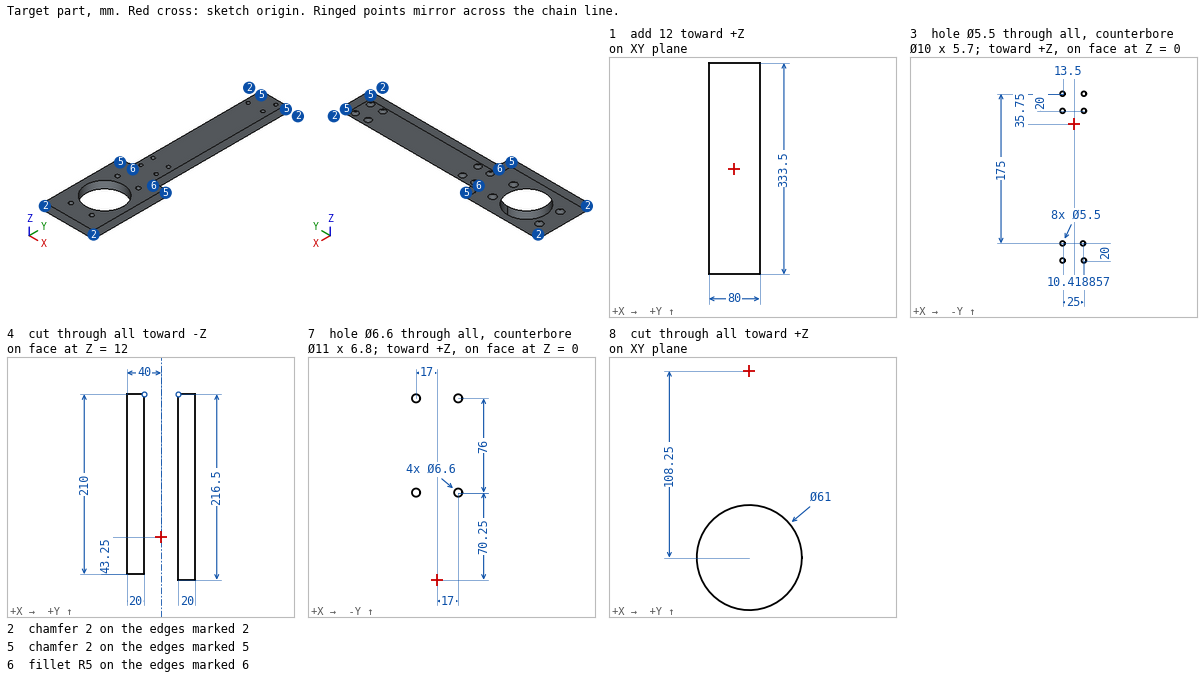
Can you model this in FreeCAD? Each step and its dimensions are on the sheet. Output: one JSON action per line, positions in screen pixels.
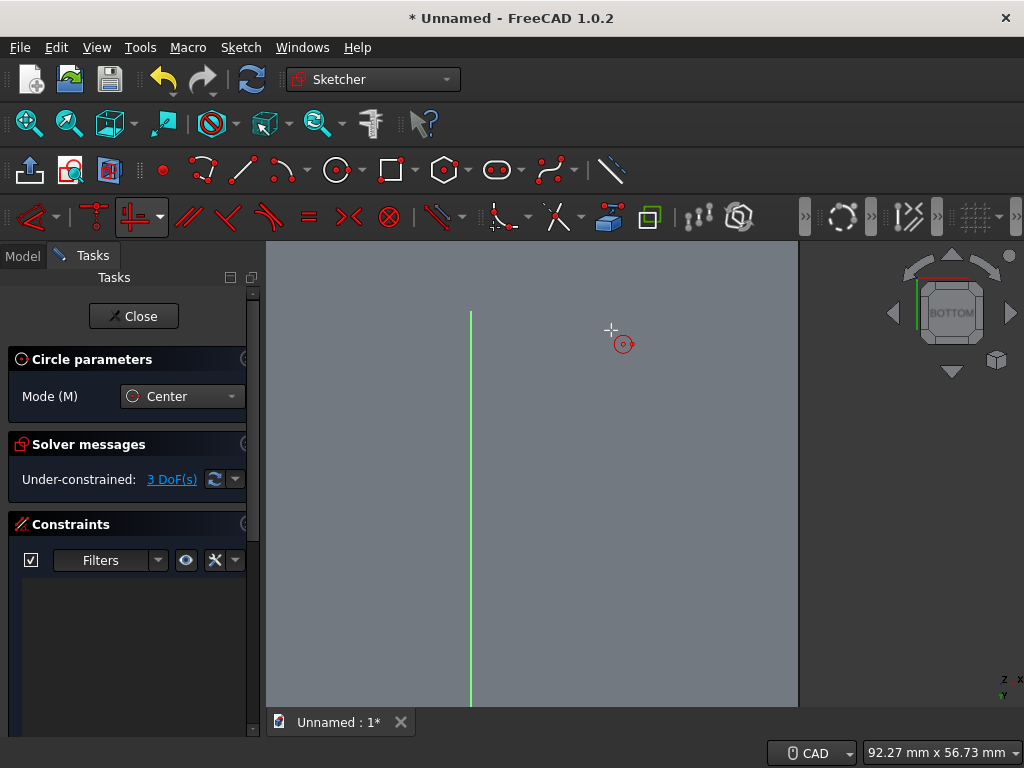
{"action": "scroll", "coordinate": [611, 329], "scroll_direction": "down", "scroll_amount": 7}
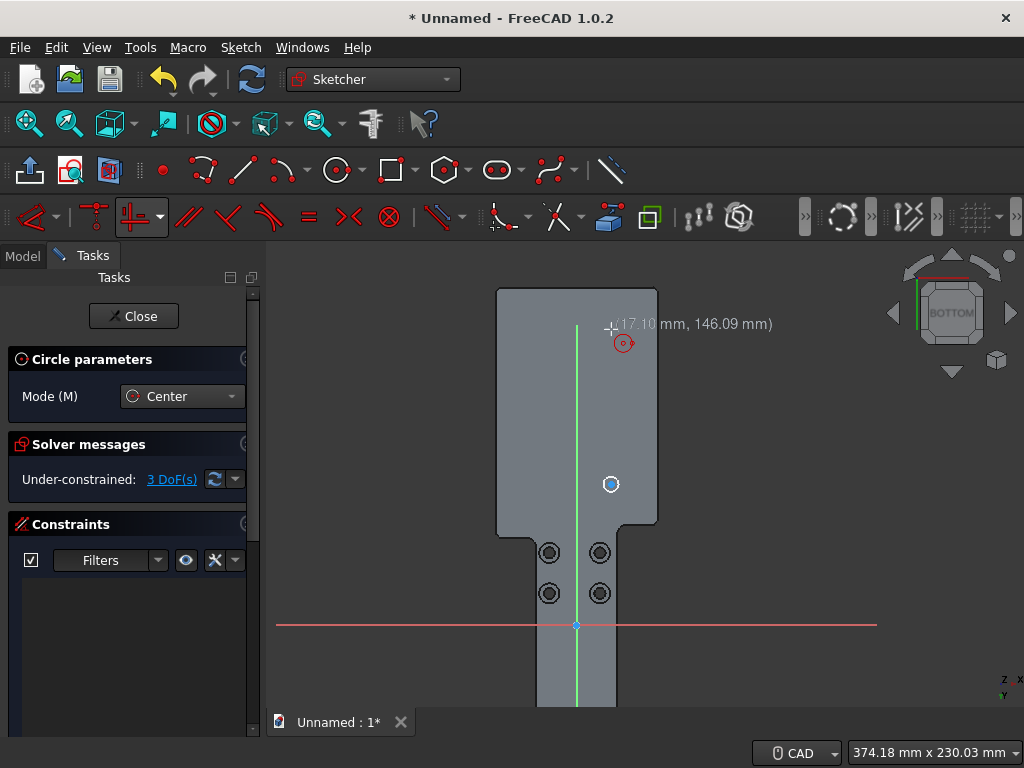
{"action": "left_click", "coordinate": [611, 329]}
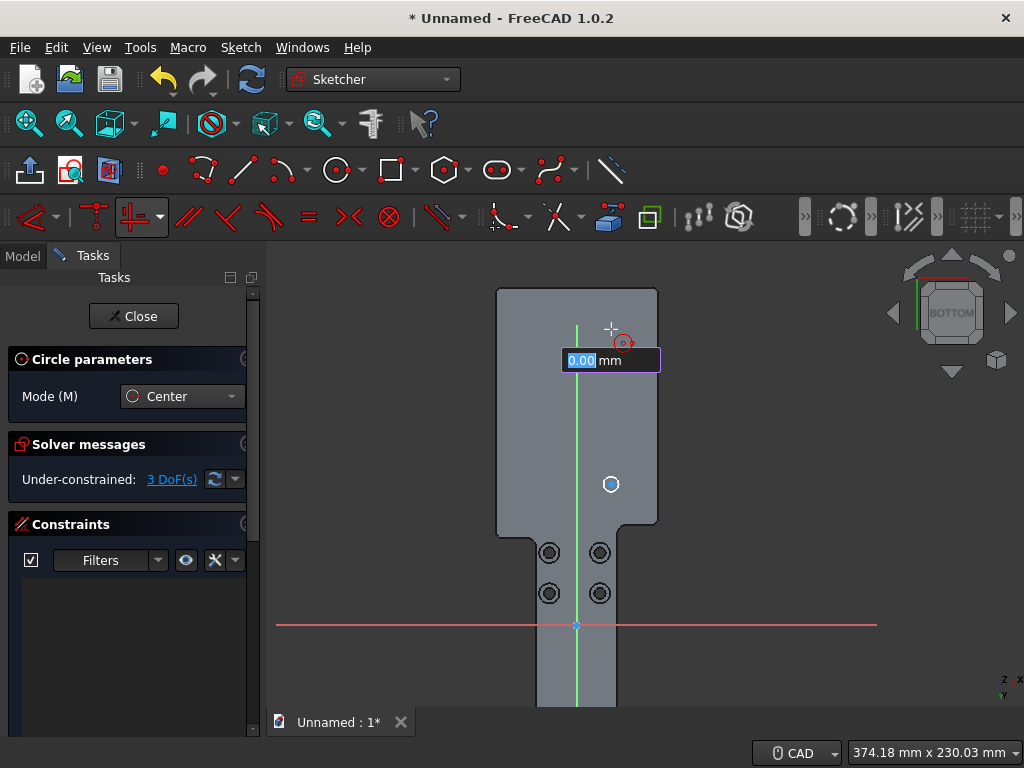
{"action": "scroll", "coordinate": [616, 324], "scroll_direction": "up", "scroll_amount": 5}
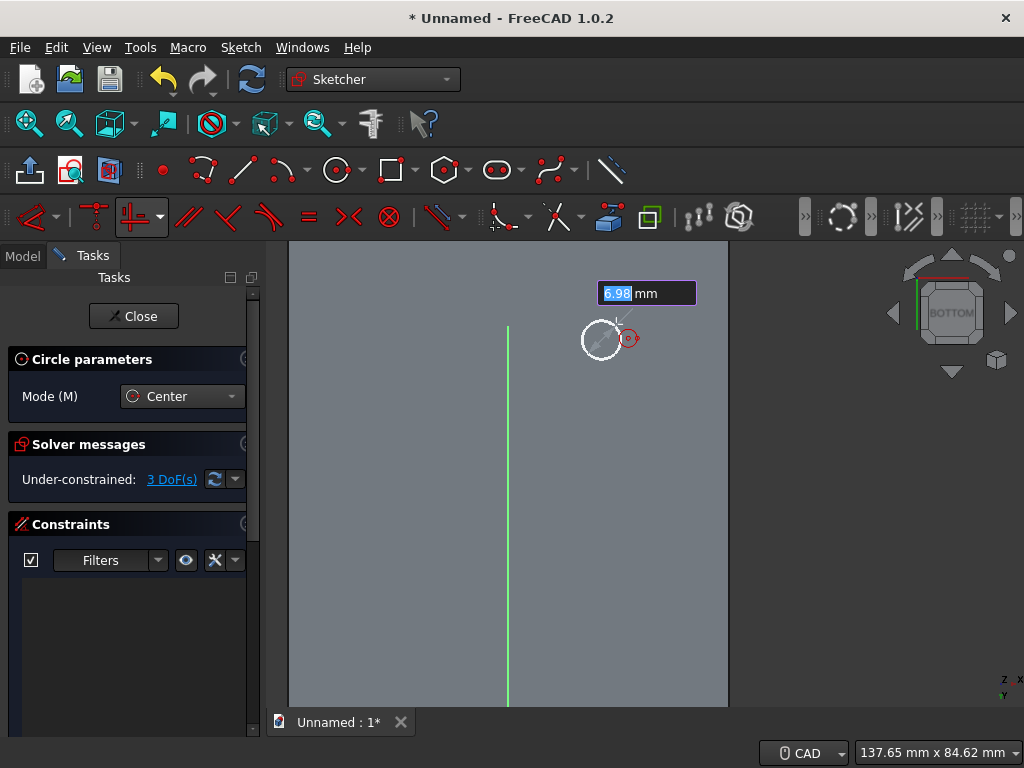
{"action": "left_click", "coordinate": [615, 325]}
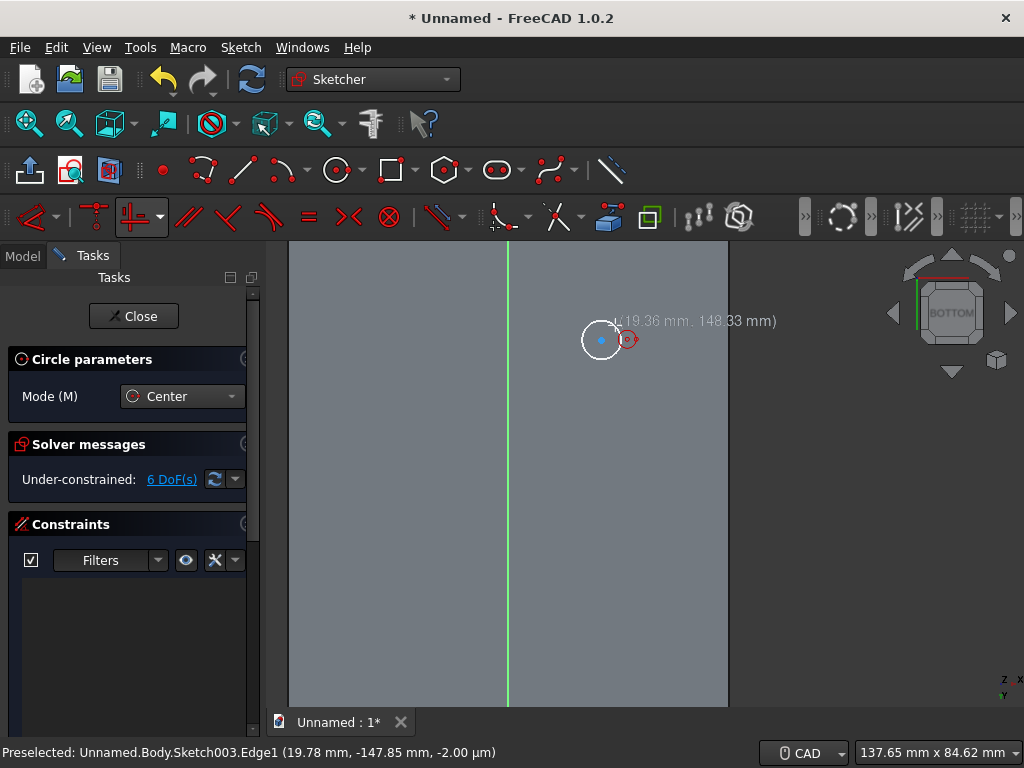
{"action": "scroll", "coordinate": [415, 337], "scroll_direction": "up", "scroll_amount": 2}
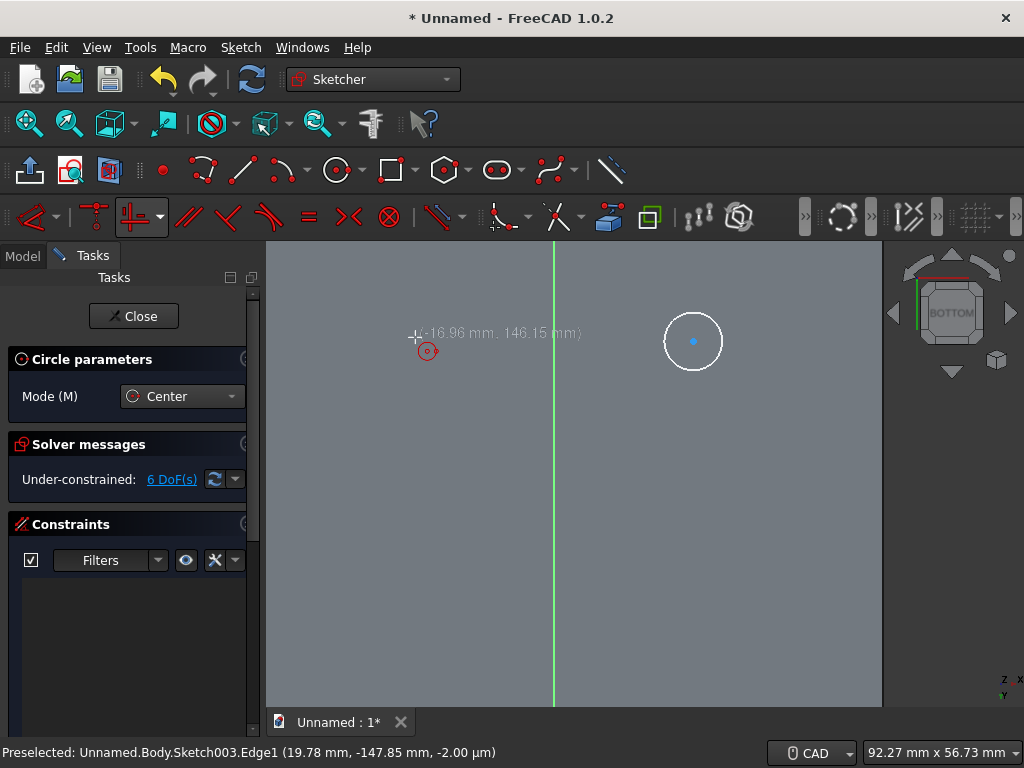
{"action": "scroll", "coordinate": [584, 326], "scroll_direction": "down", "scroll_amount": 7}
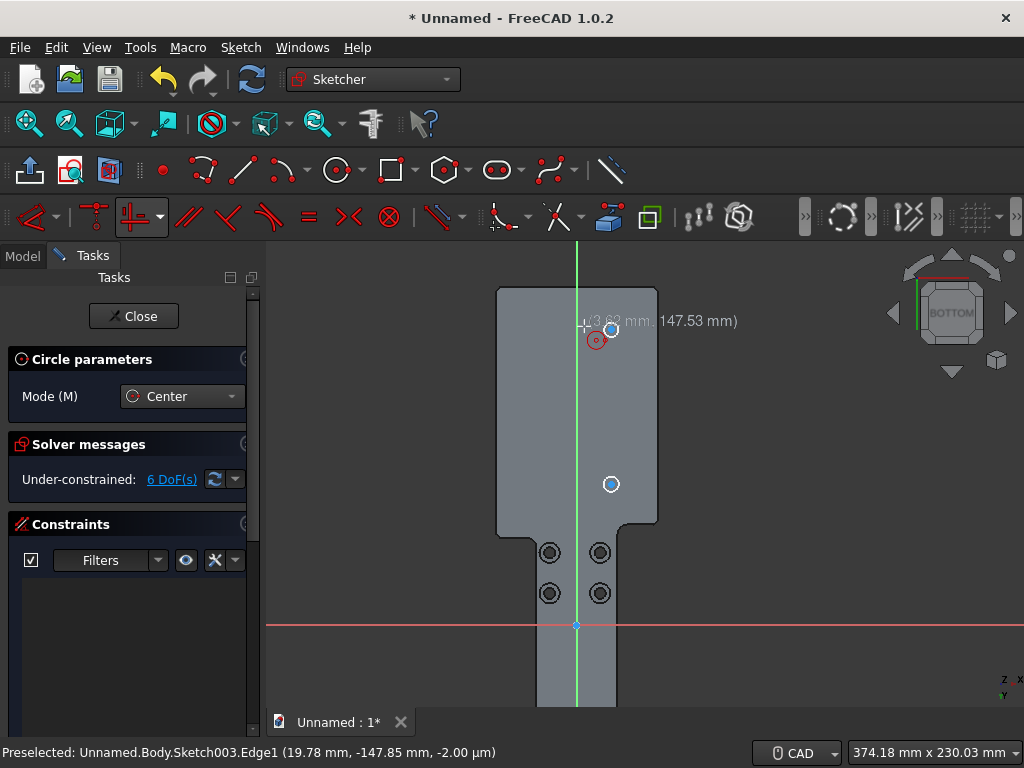
{"action": "left_click", "coordinate": [543, 329]}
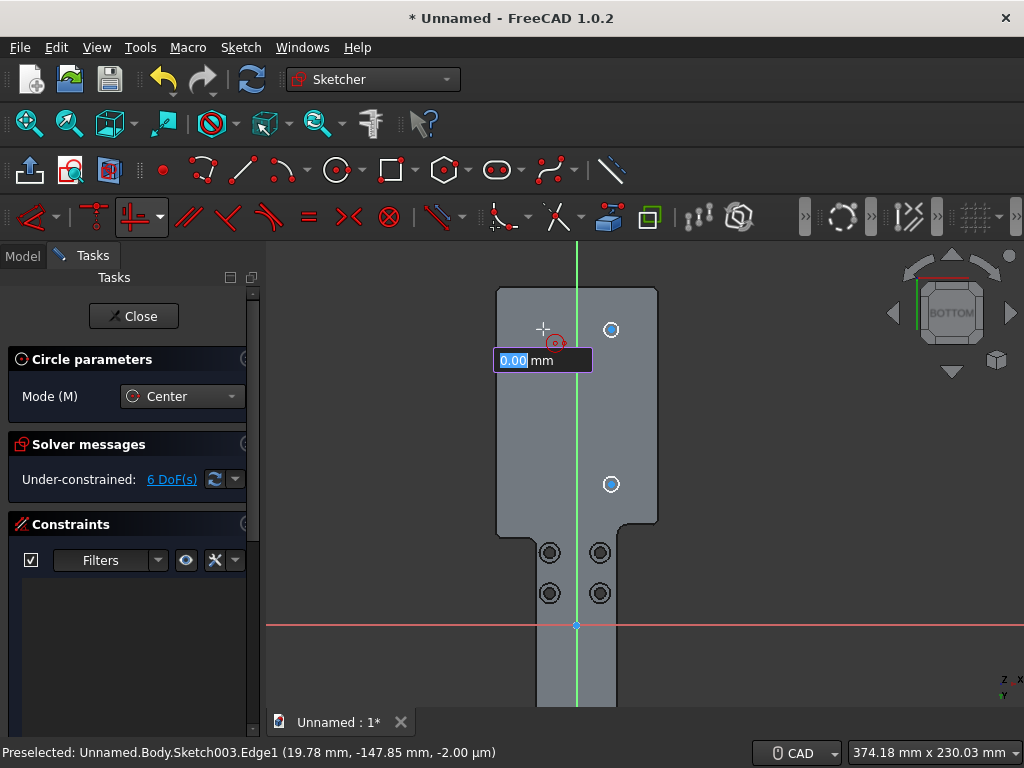
{"action": "scroll", "coordinate": [547, 324], "scroll_direction": "up", "scroll_amount": 5}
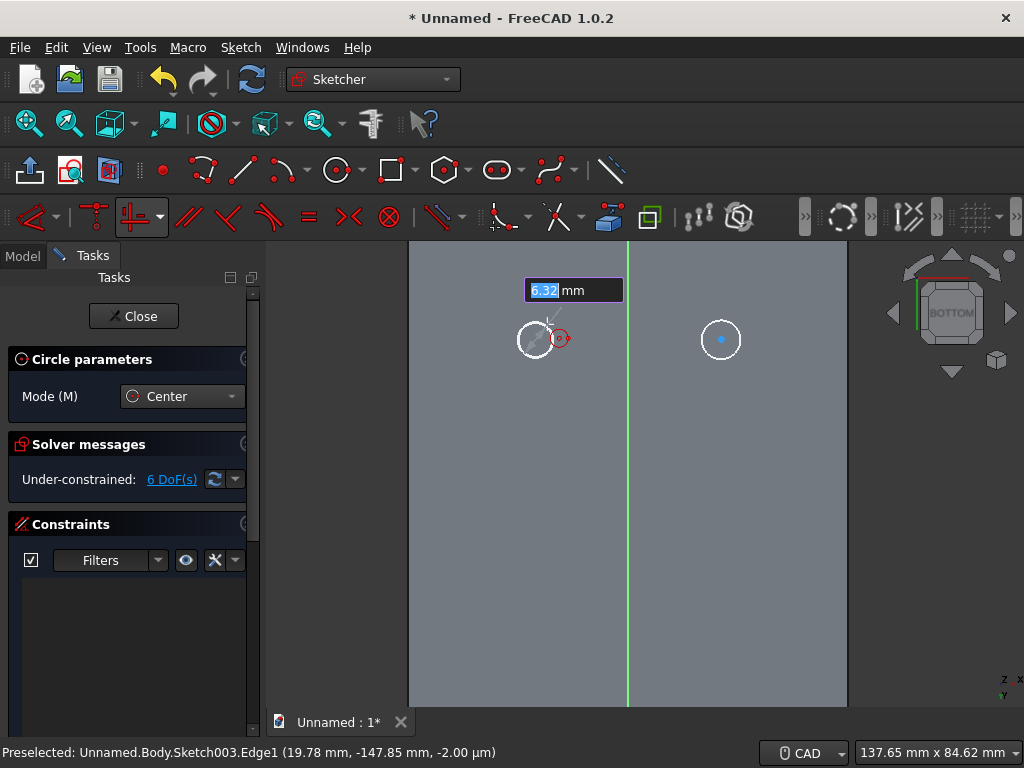
{"action": "left_click", "coordinate": [547, 324]}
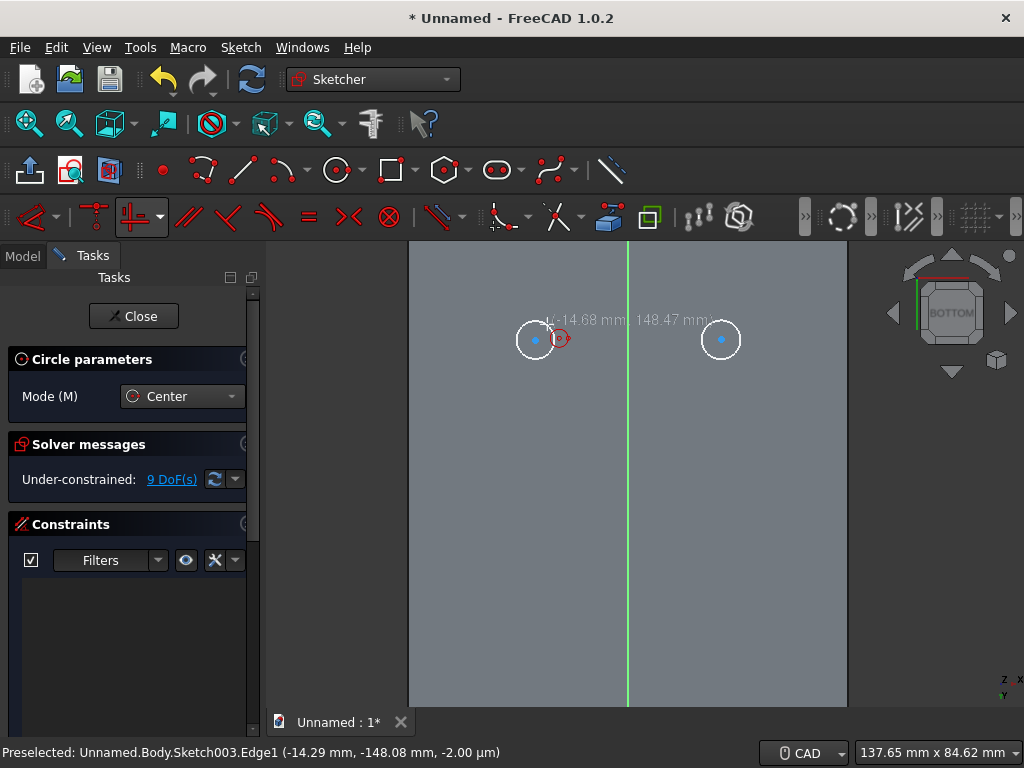
{"action": "scroll", "coordinate": [547, 325], "scroll_direction": "down", "scroll_amount": 5}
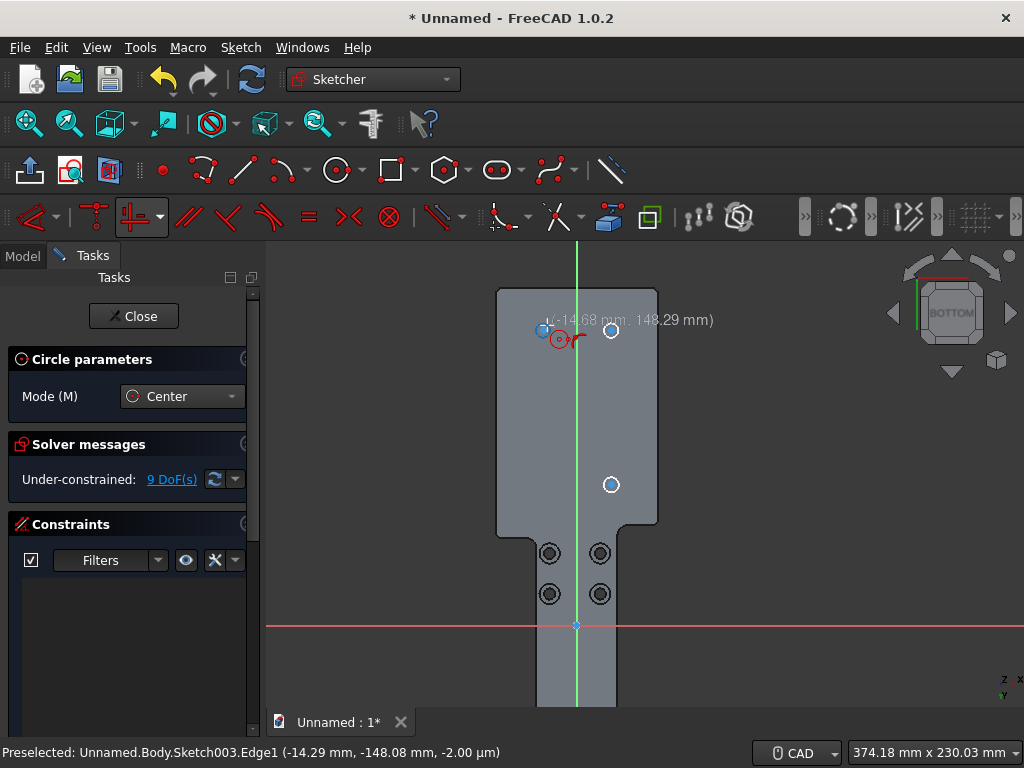
{"action": "scroll", "coordinate": [543, 484], "scroll_direction": "up", "scroll_amount": 7}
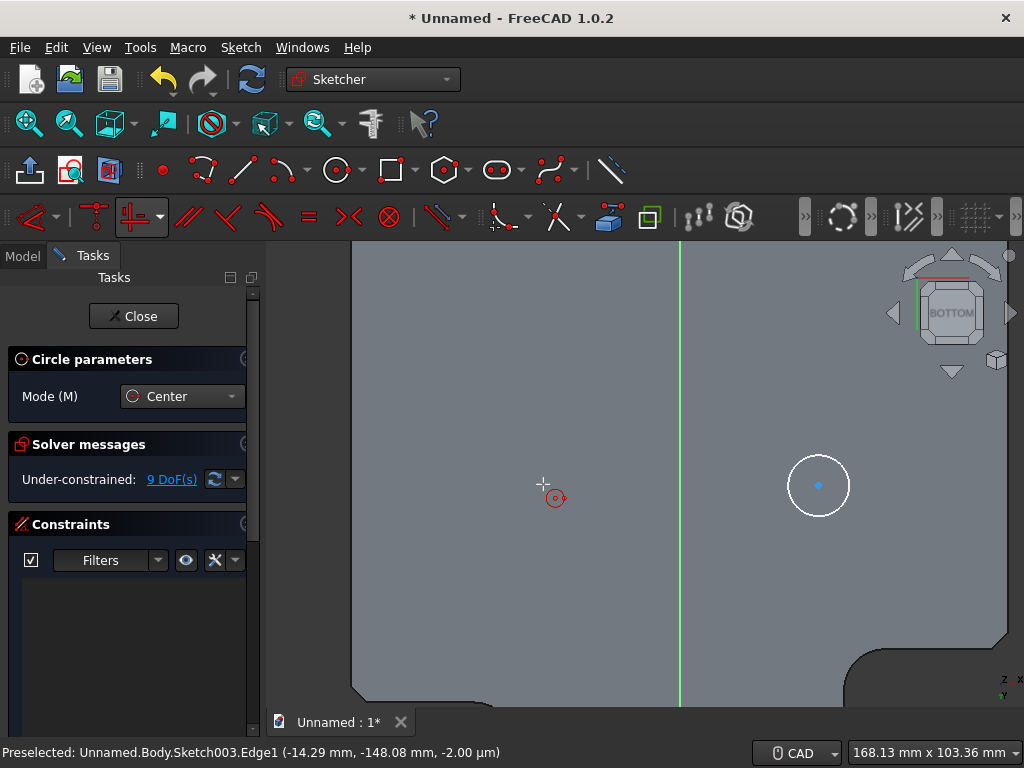
{"action": "scroll", "coordinate": [543, 484], "scroll_direction": "down", "scroll_amount": 7}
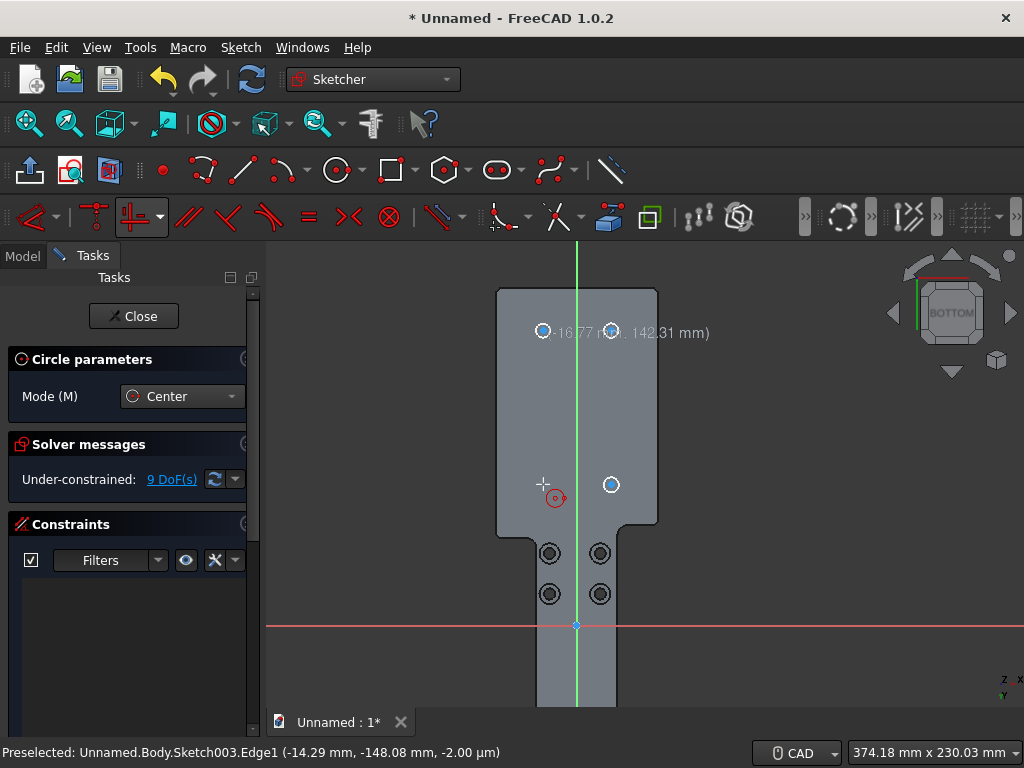
{"action": "left_click", "coordinate": [543, 484]}